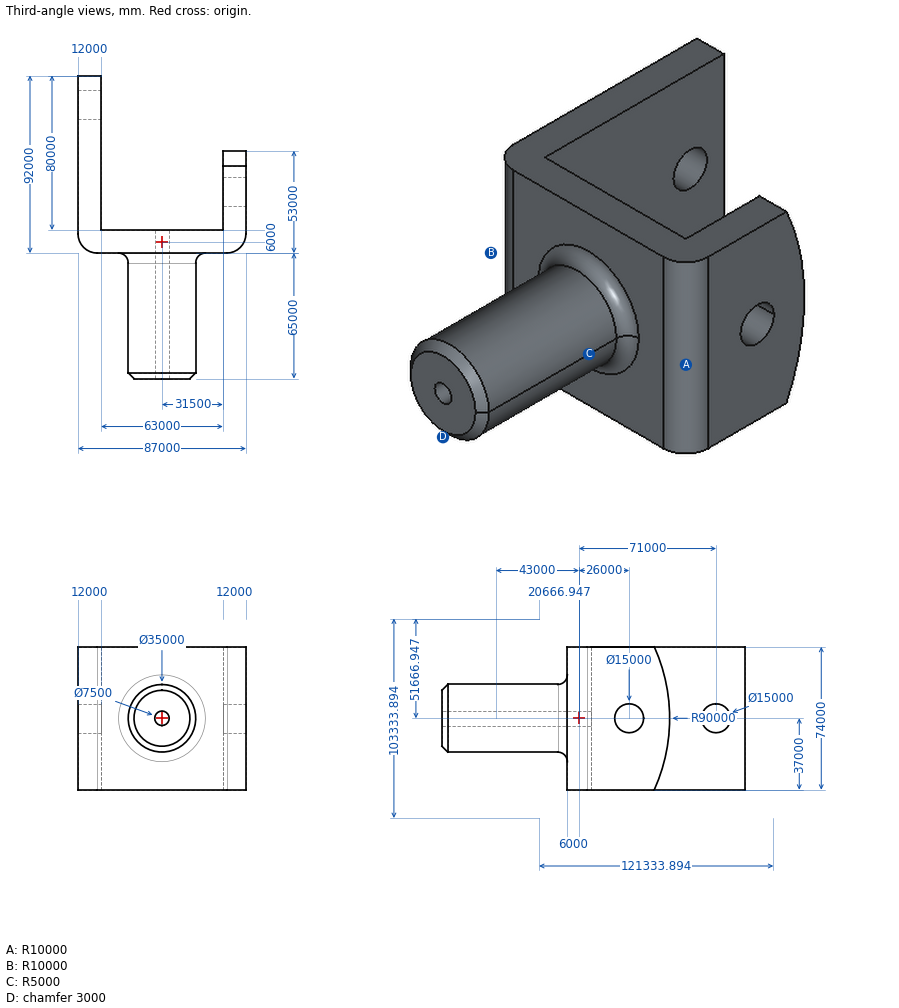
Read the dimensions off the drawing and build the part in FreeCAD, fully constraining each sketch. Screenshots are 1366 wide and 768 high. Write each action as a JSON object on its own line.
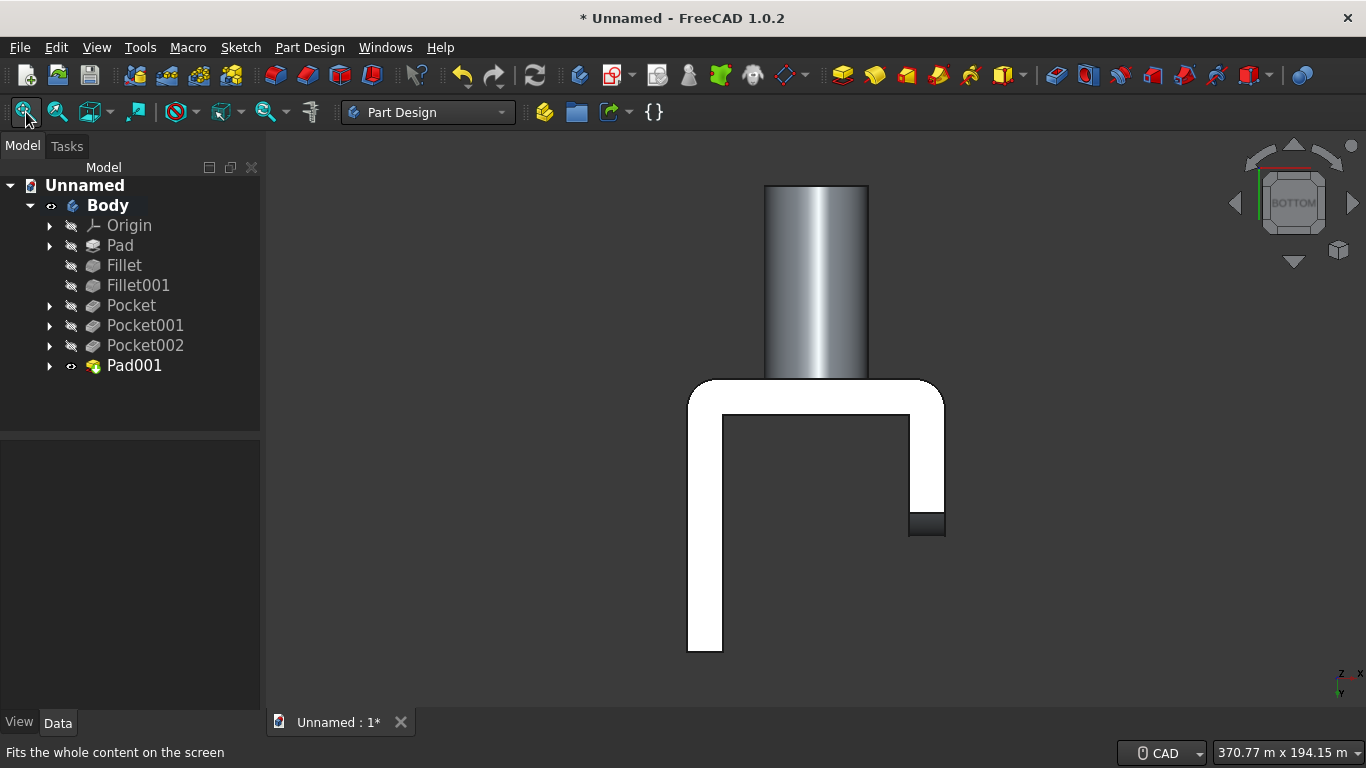
{"action": "key", "text": "4"}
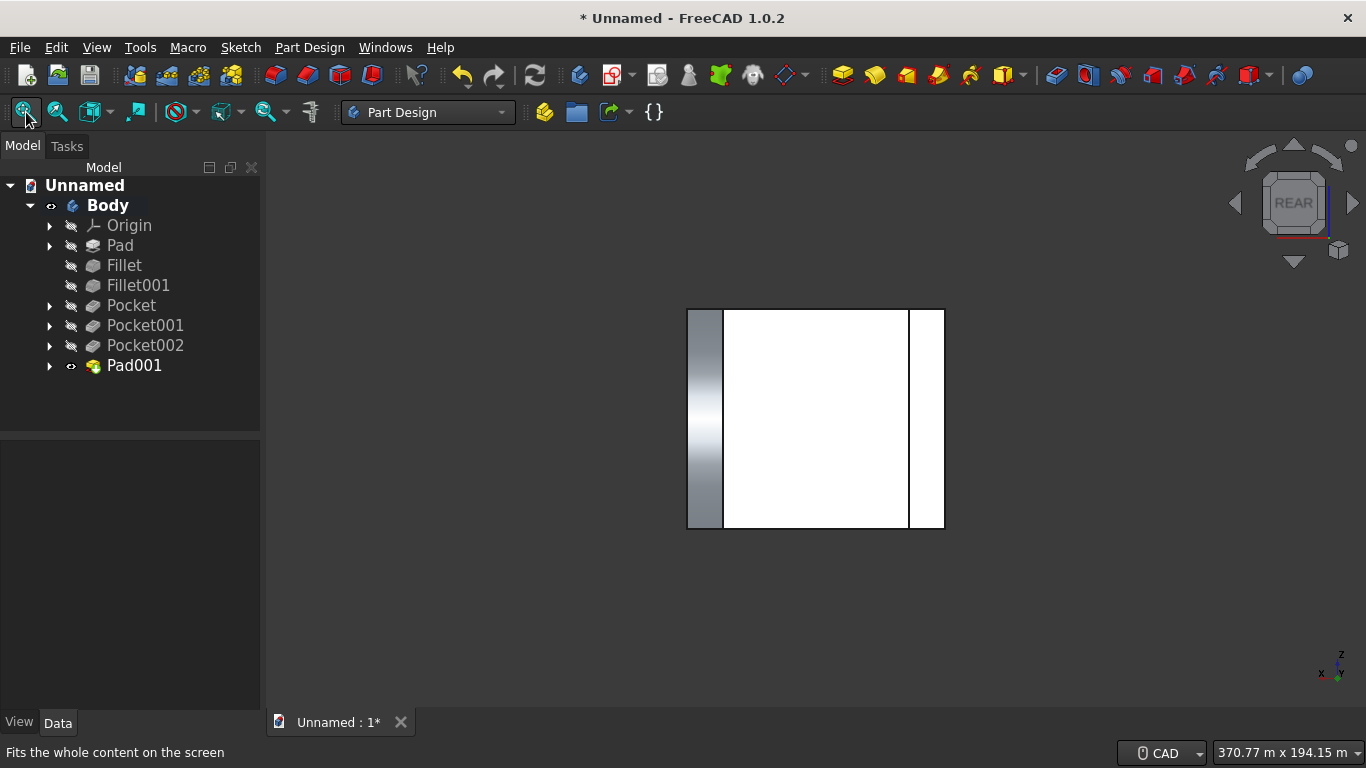
{"action": "left_click", "coordinate": [26, 112]}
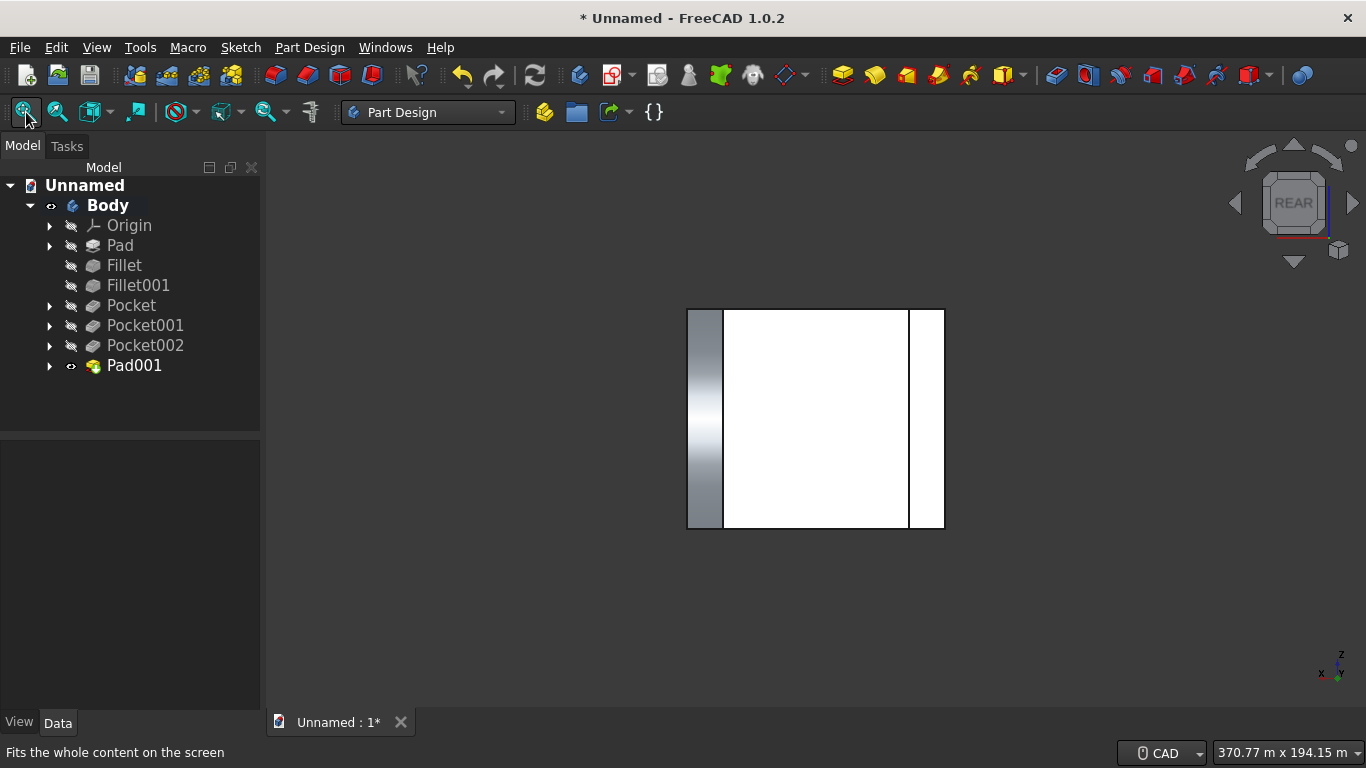
{"action": "key", "text": "6"}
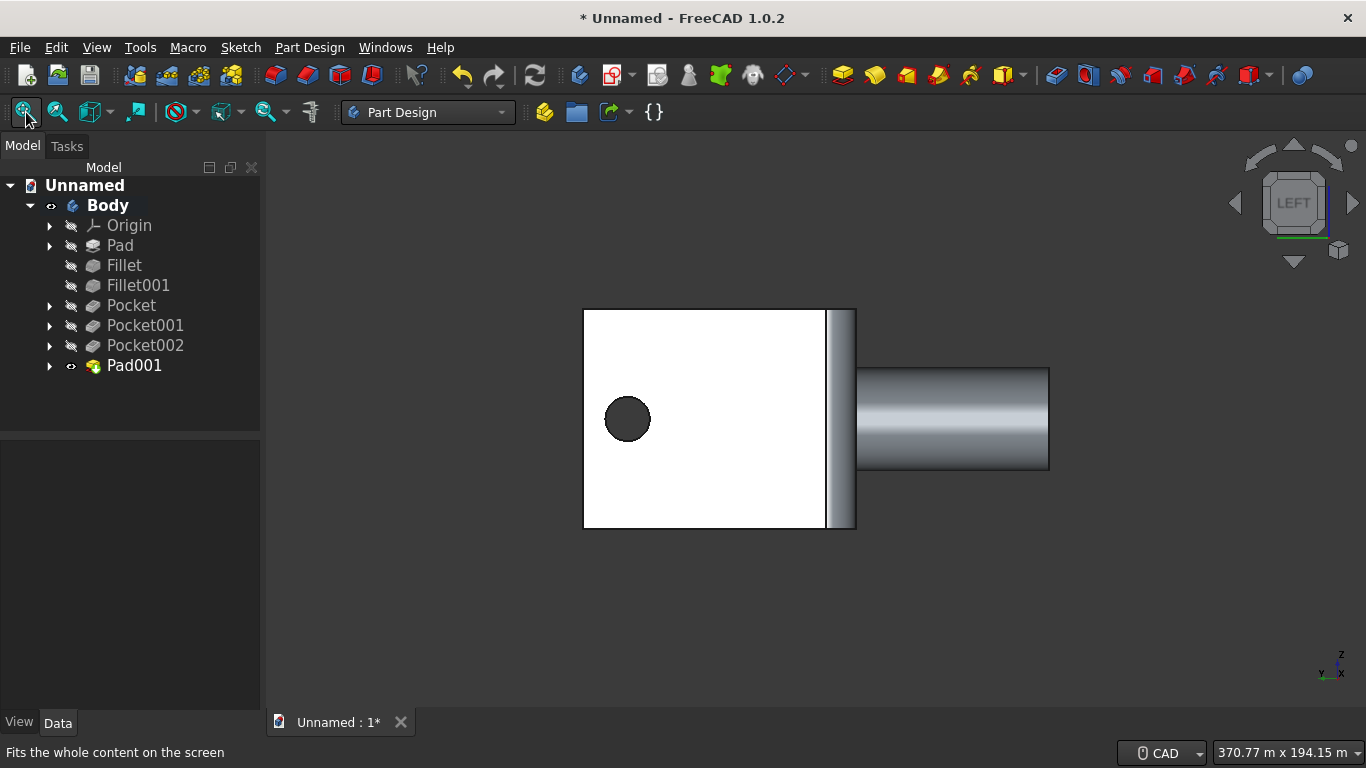
{"action": "left_click", "coordinate": [26, 112]}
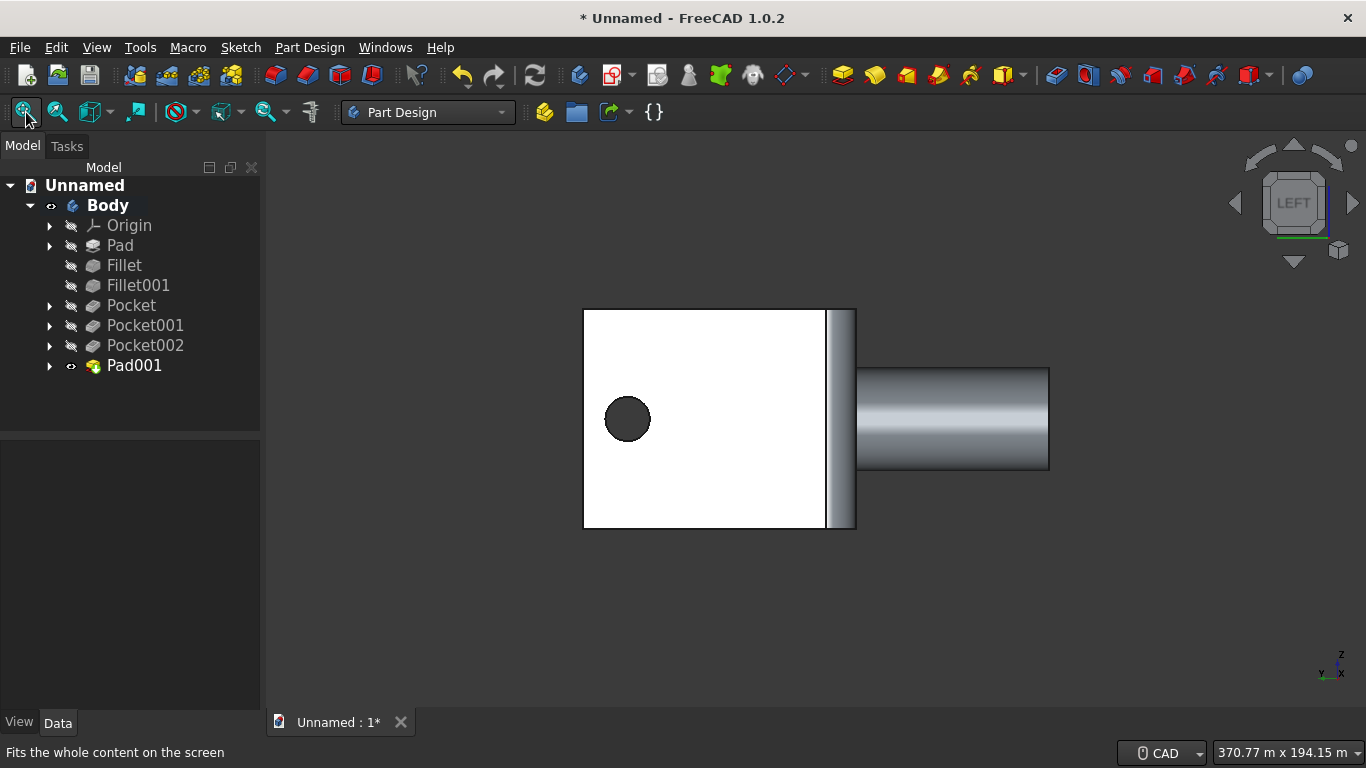
{"action": "key", "text": "v 3"}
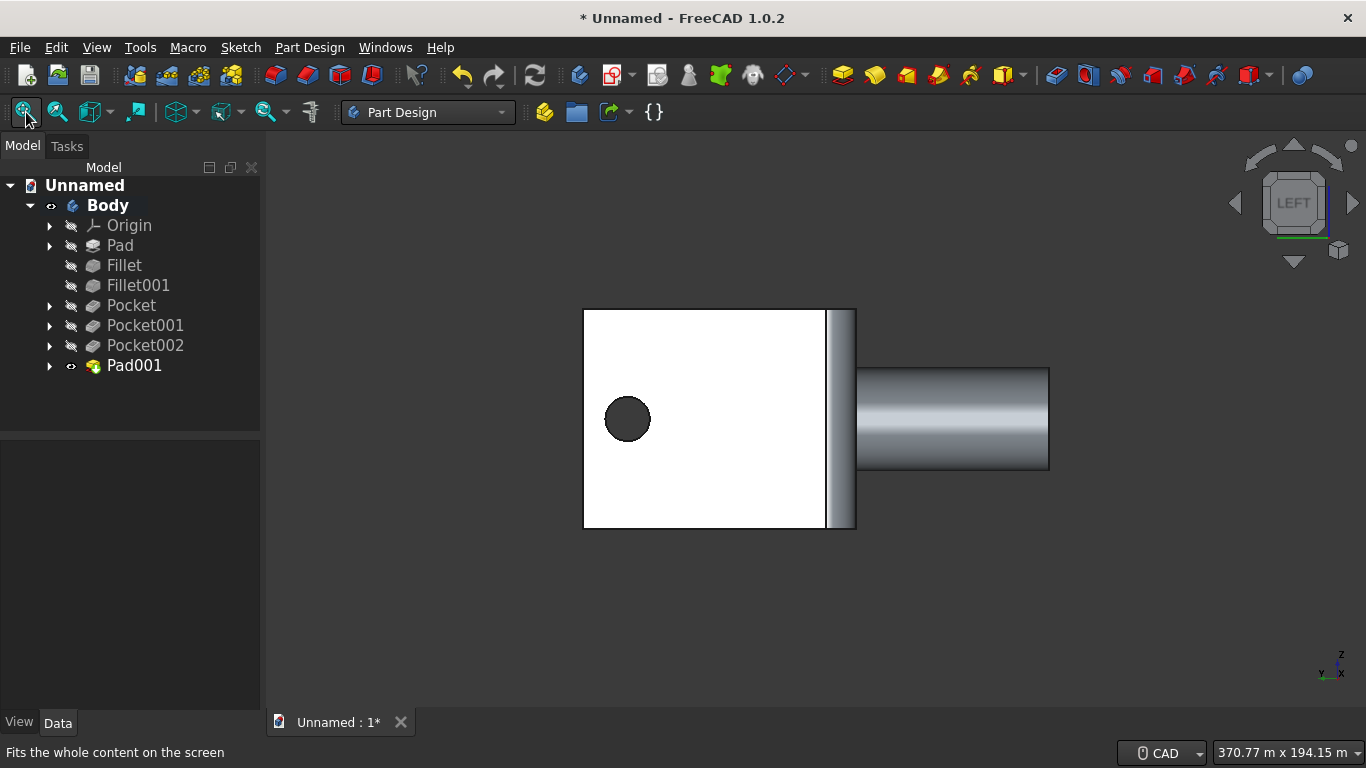
{"action": "key", "text": "0"}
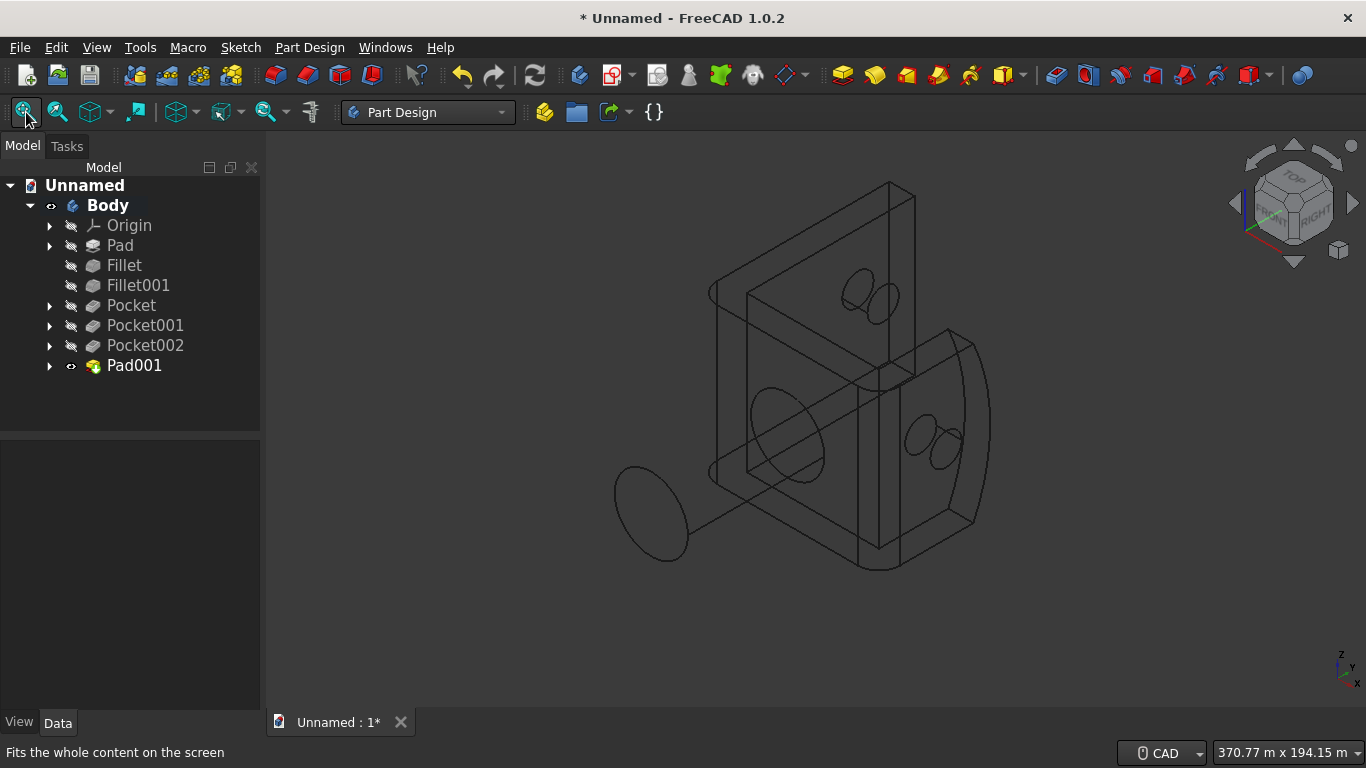
{"action": "left_click", "coordinate": [751, 413]}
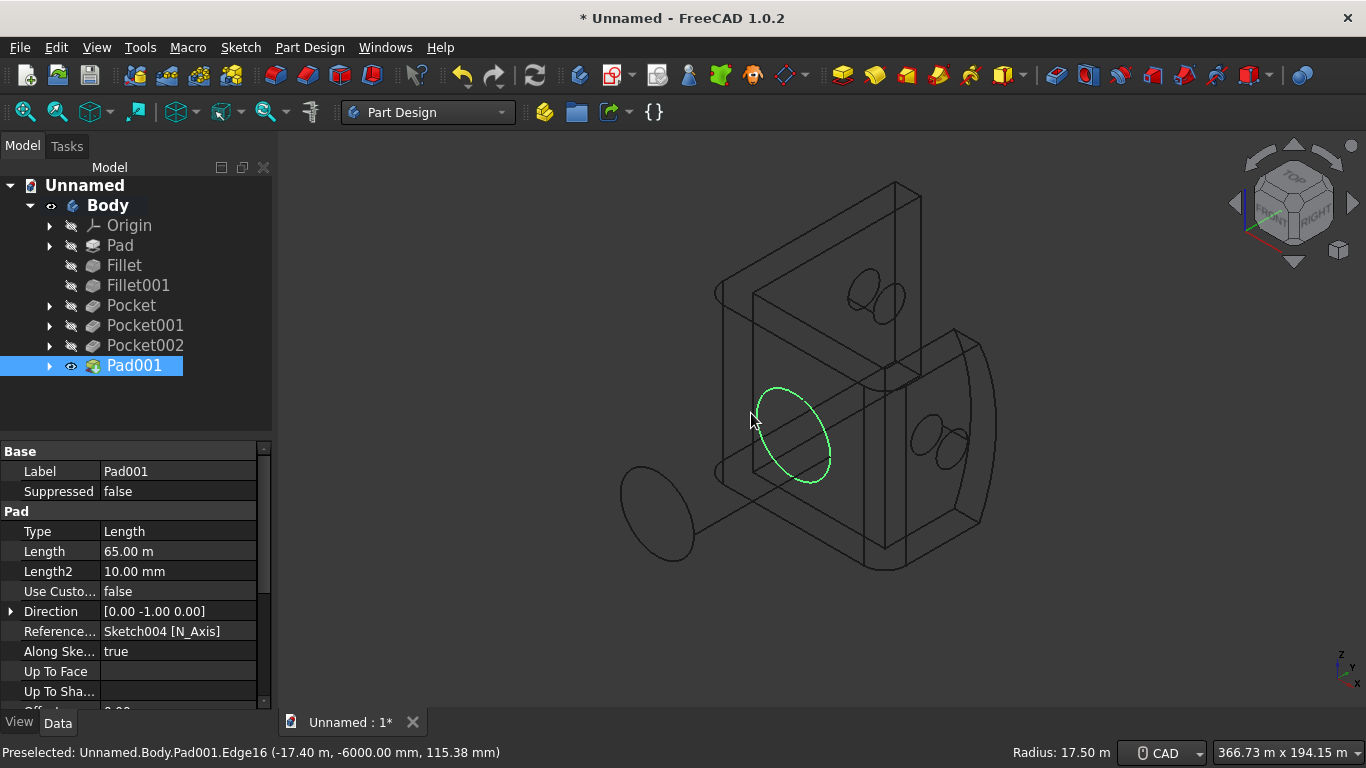
{"action": "key", "text": "v 1"}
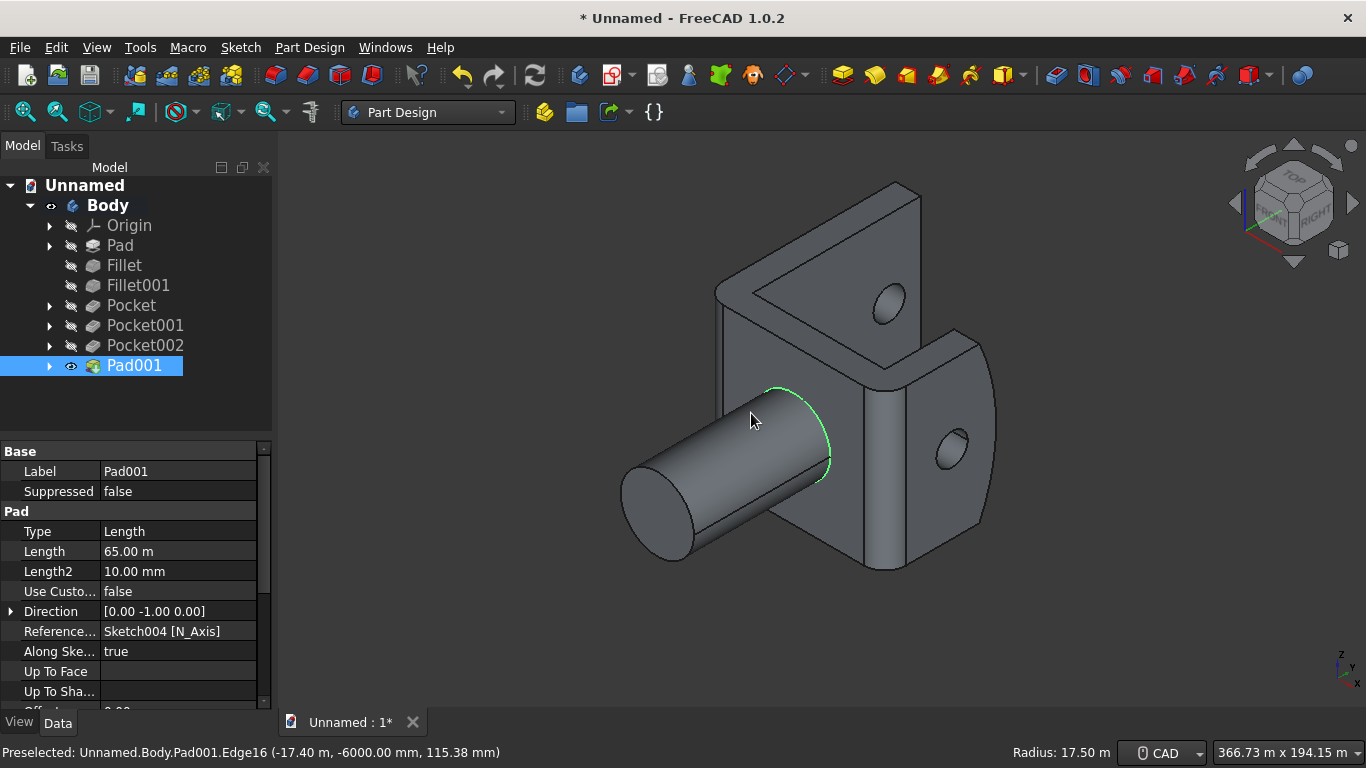
{"action": "left_click", "coordinate": [276, 76]}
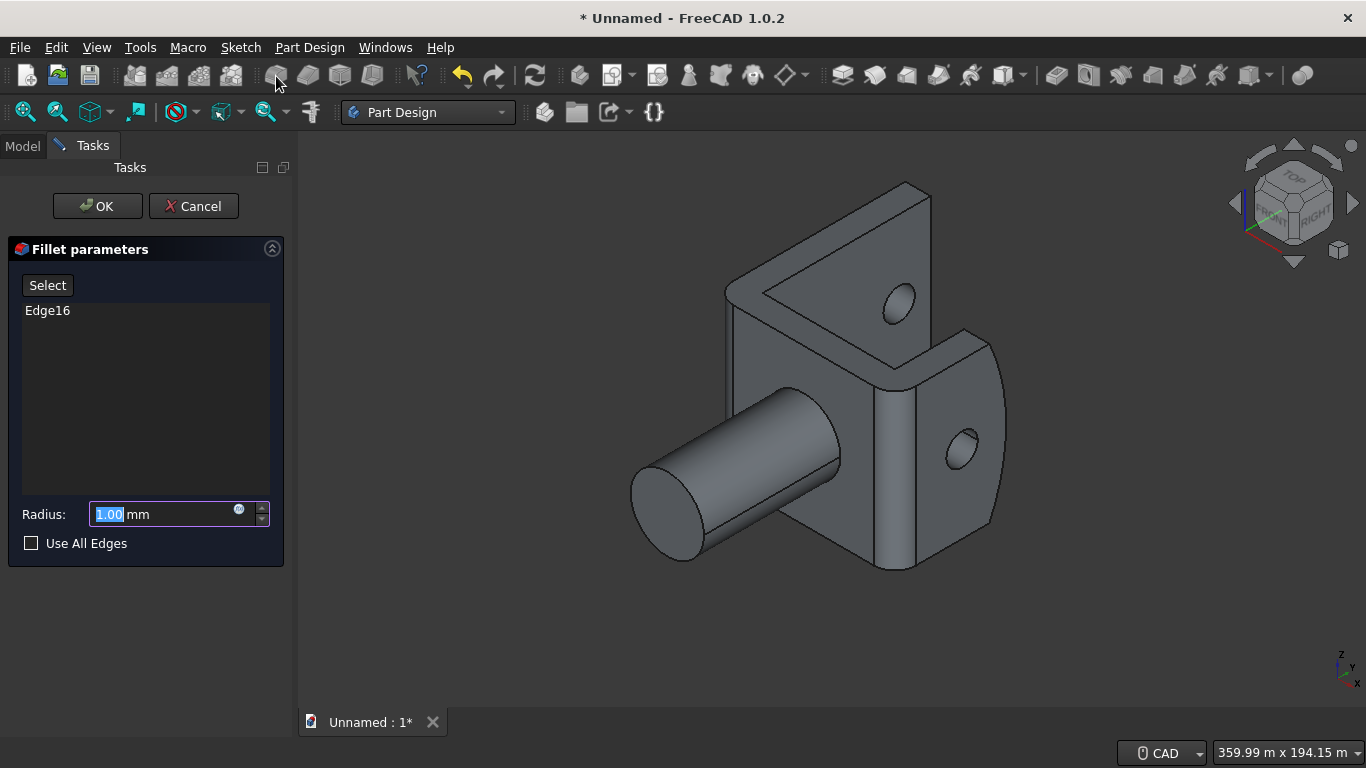
{"action": "type", "text": "5000"}
{"action": "key", "text": "Tab"}